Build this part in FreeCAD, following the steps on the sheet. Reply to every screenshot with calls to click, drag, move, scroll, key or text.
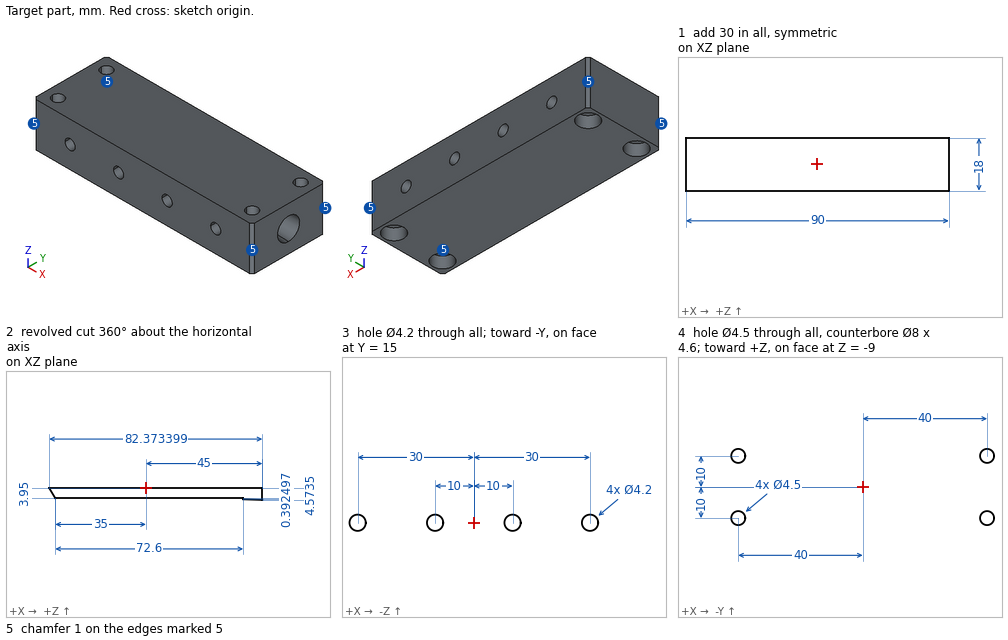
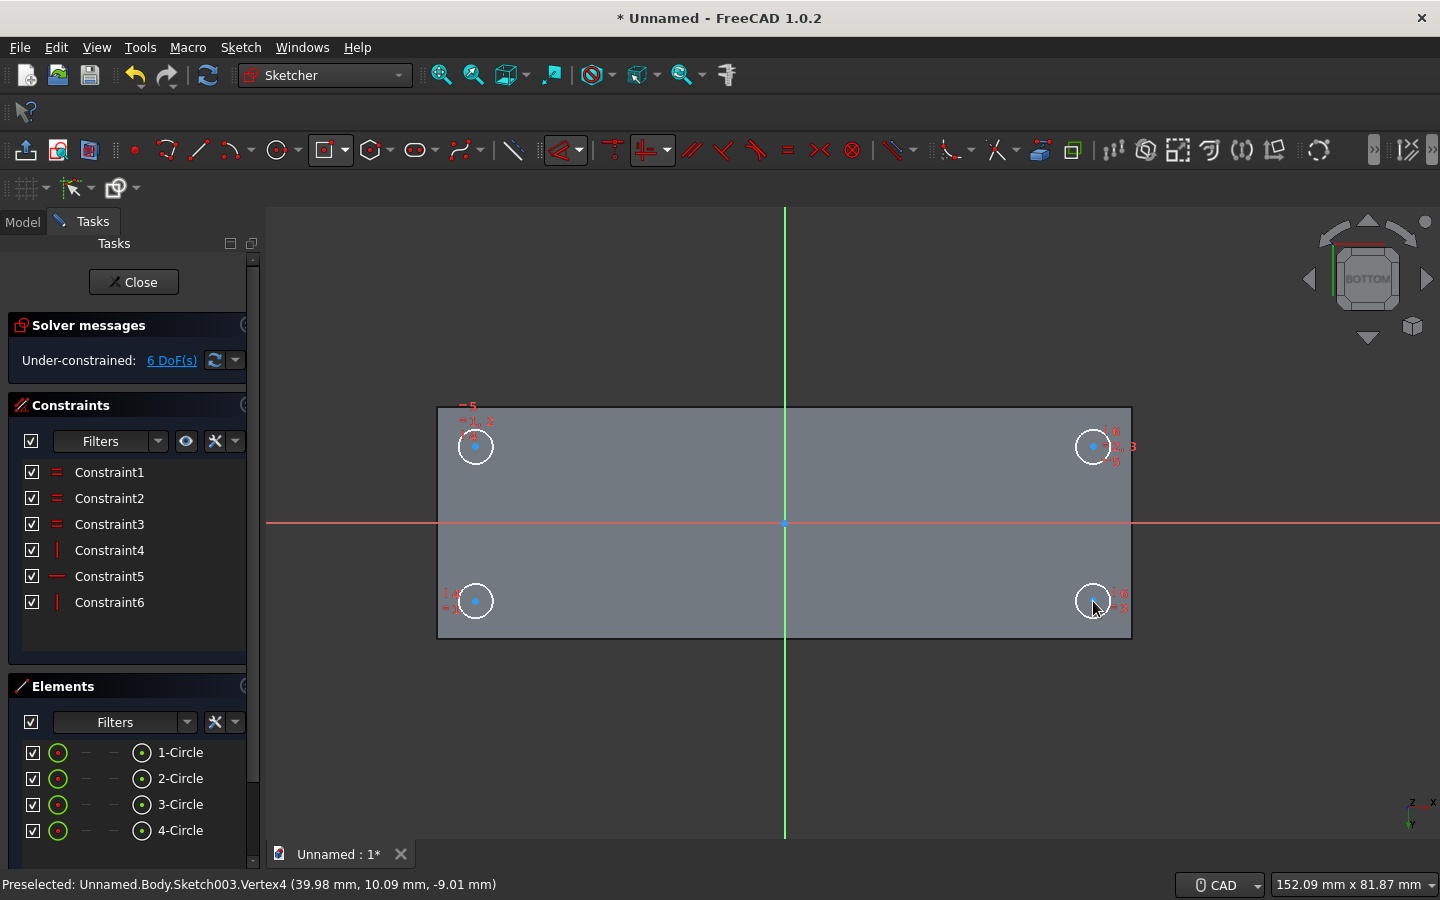
click(476, 601)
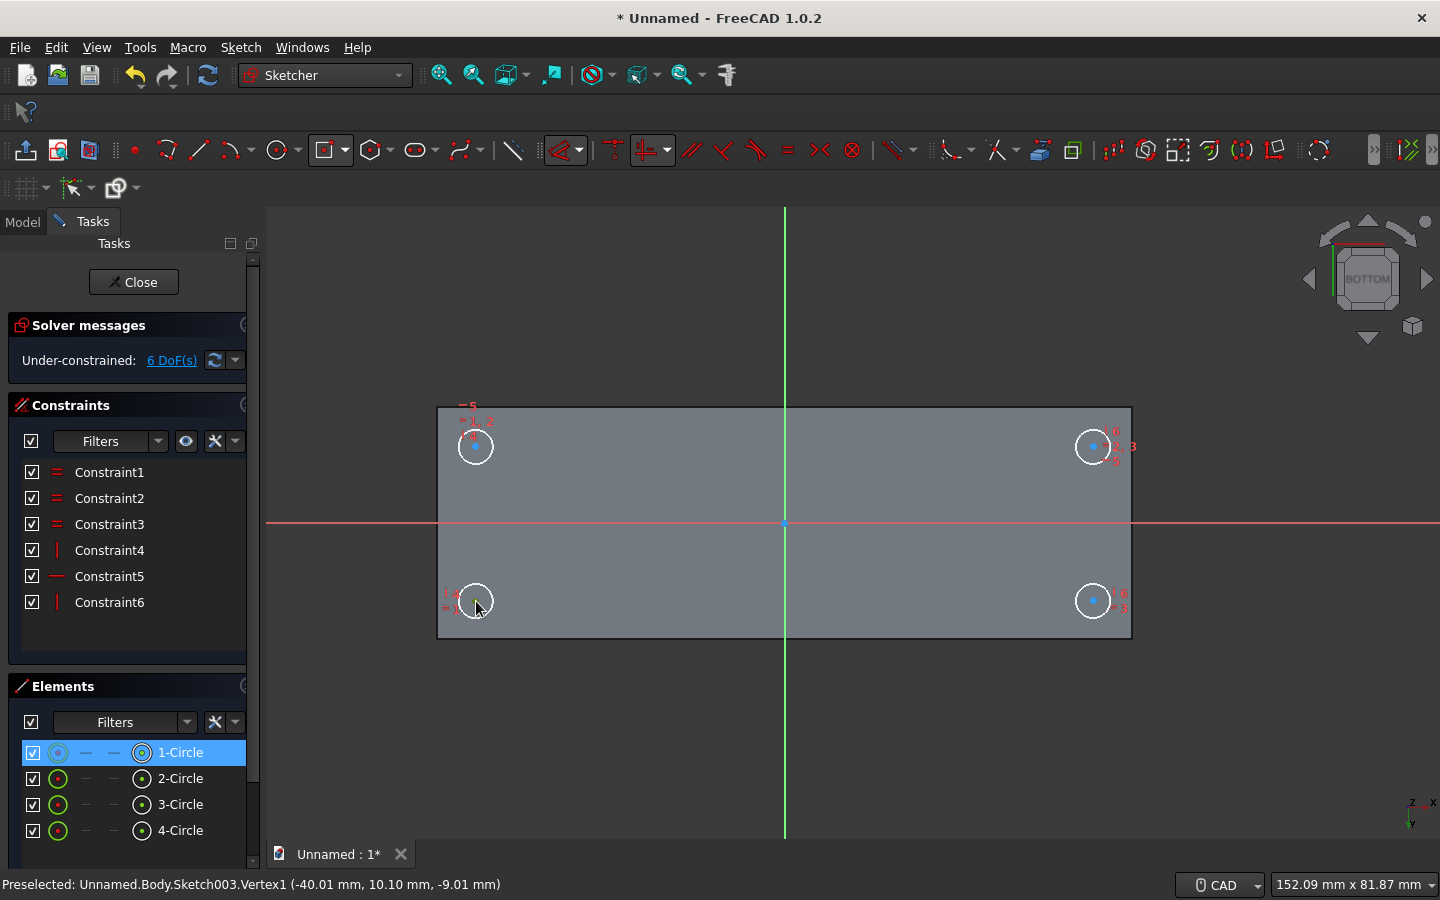
click(1093, 601)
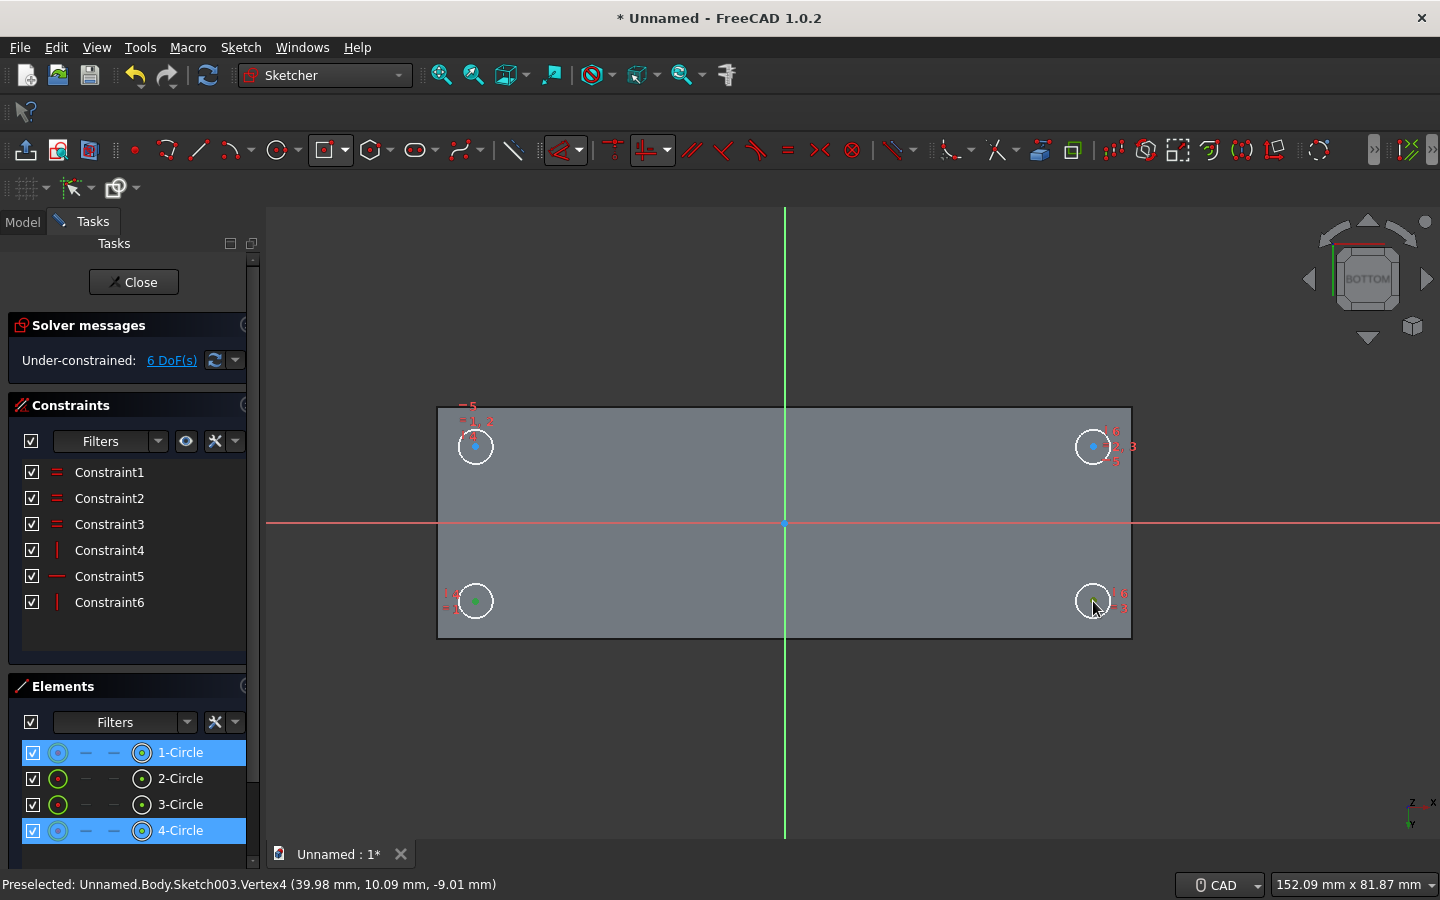
click(670, 150)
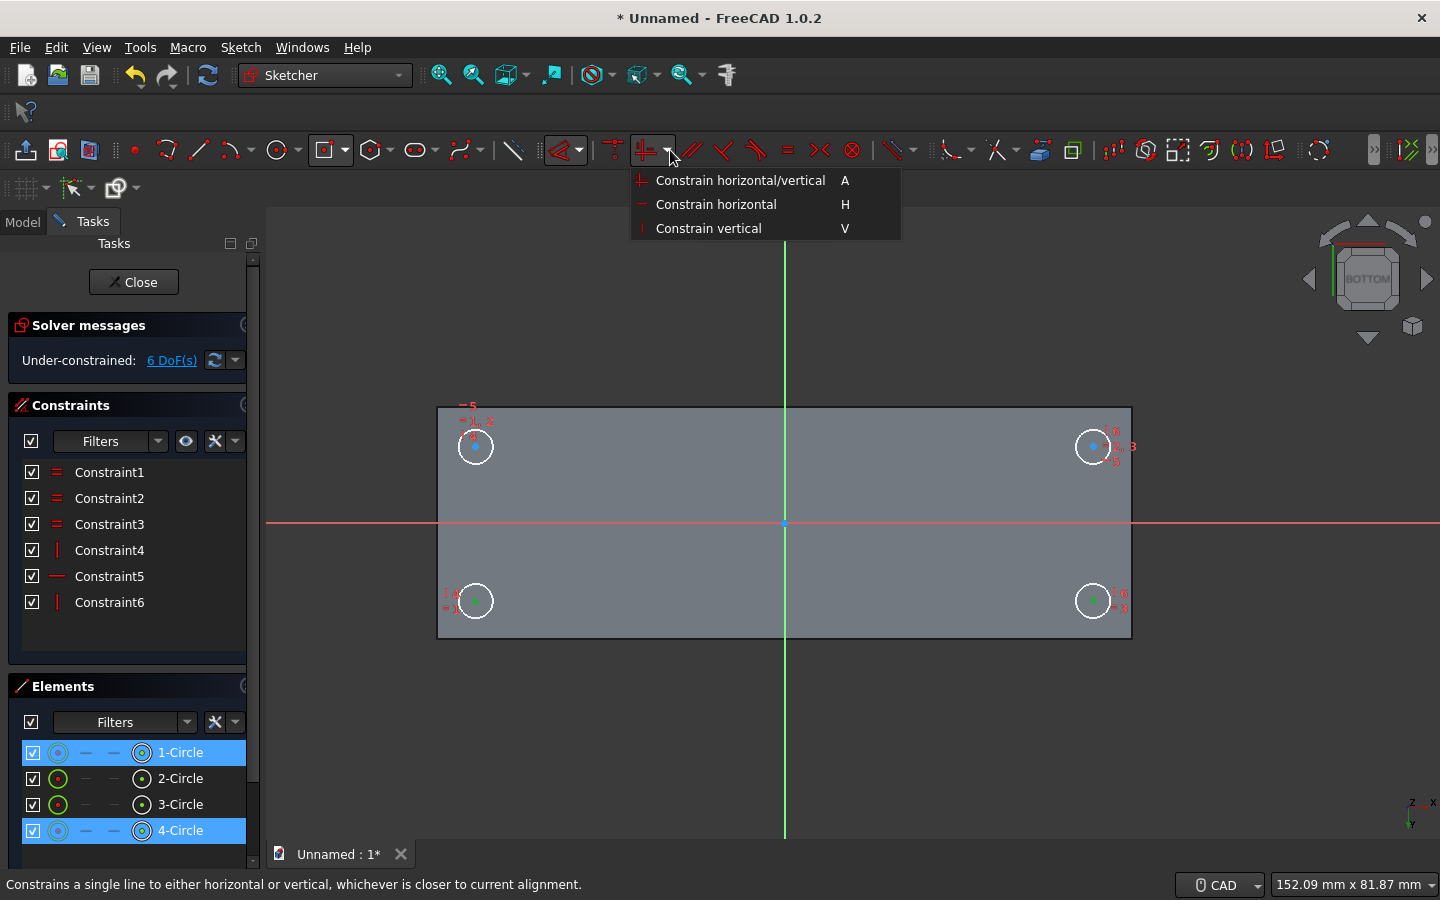
click(766, 204)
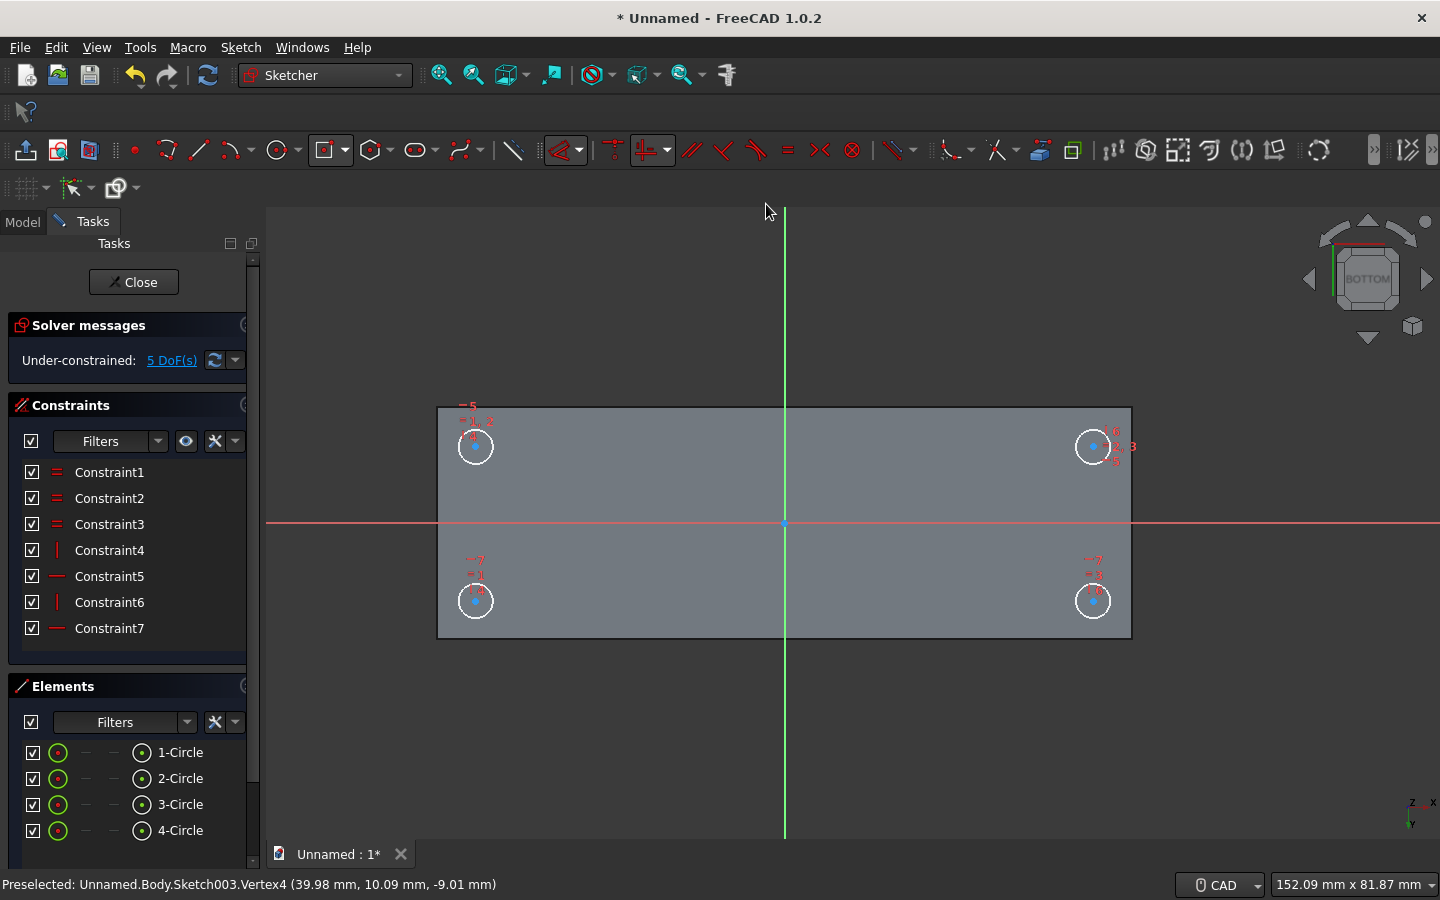
click(488, 589)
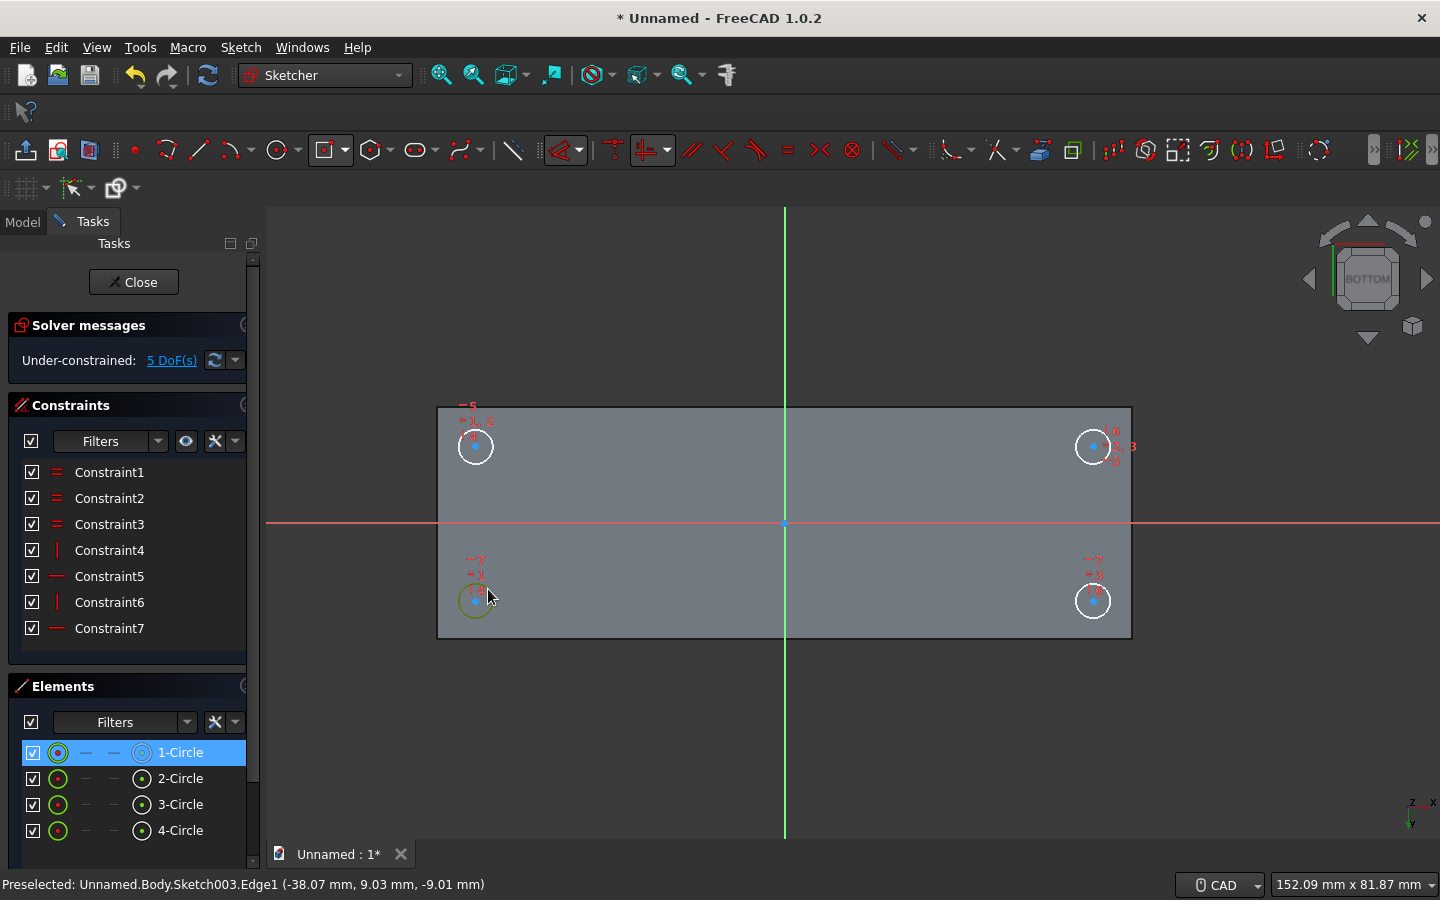
key(k)
key(o)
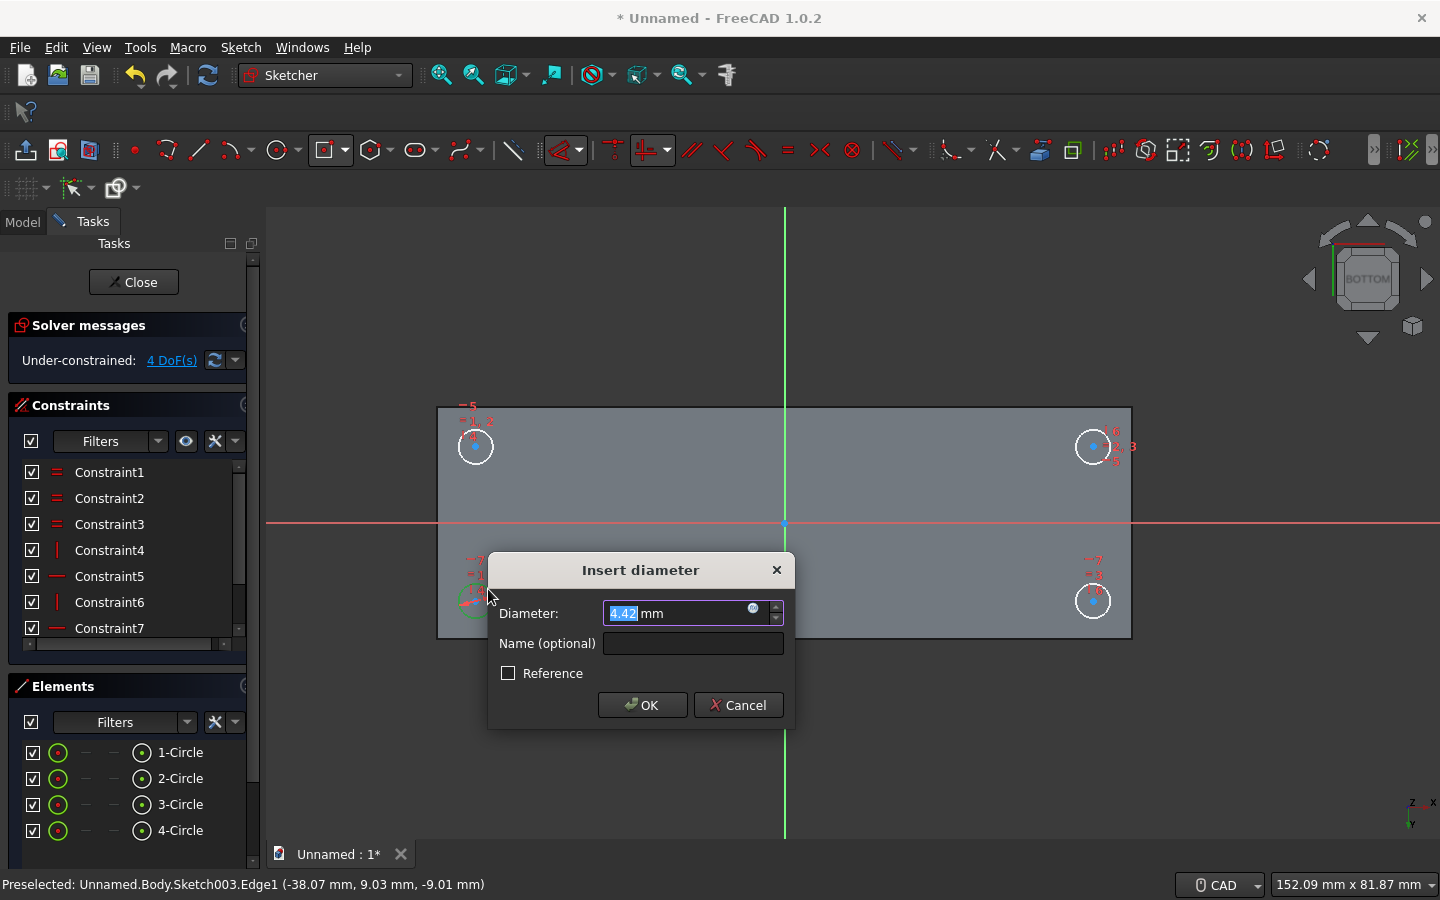
text(4.5)
key(Return)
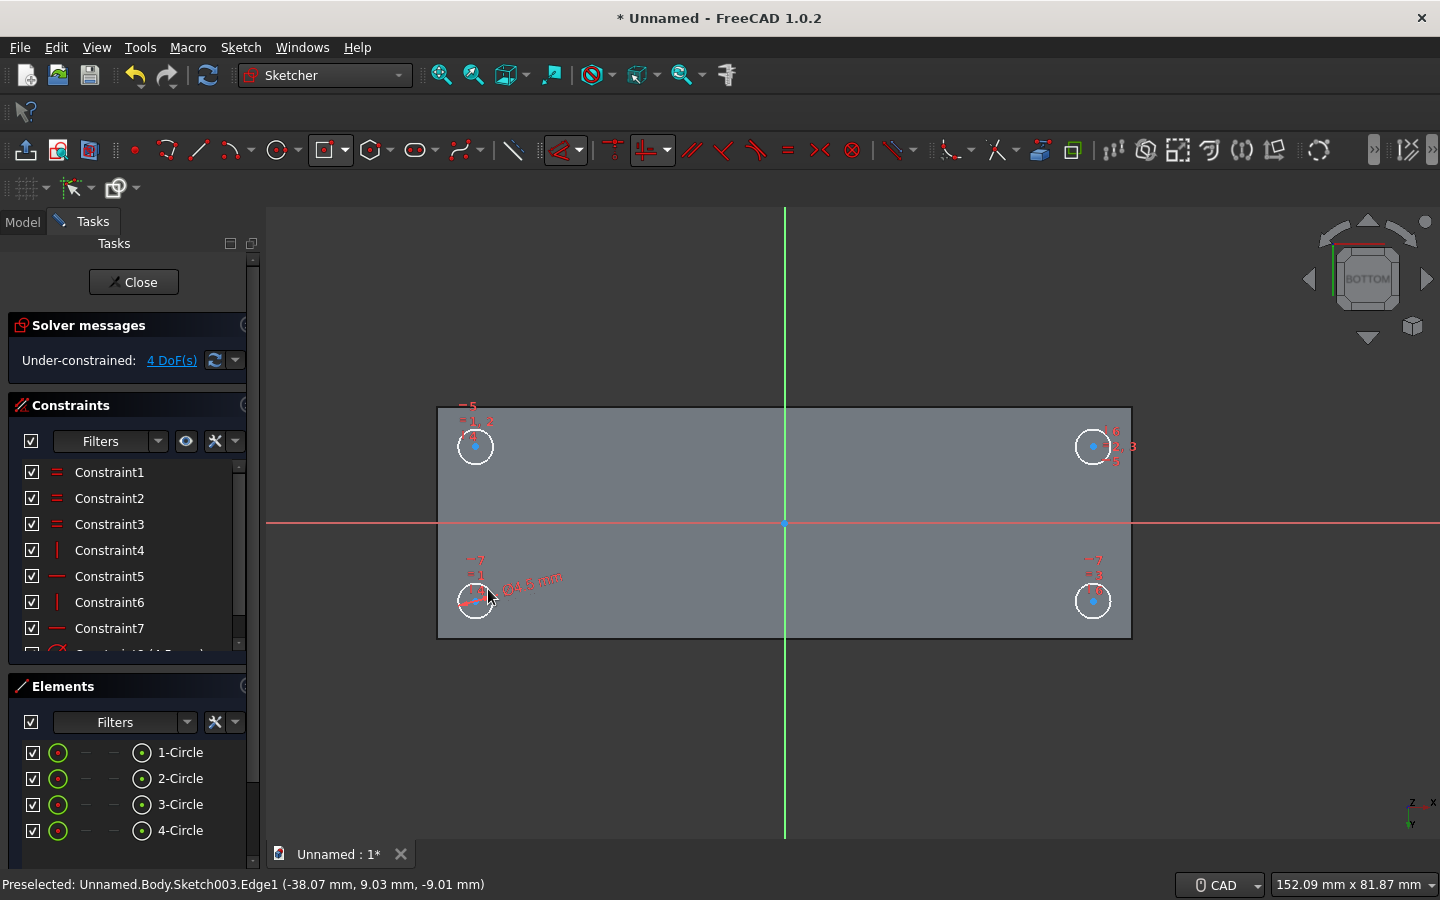
click(476, 601)